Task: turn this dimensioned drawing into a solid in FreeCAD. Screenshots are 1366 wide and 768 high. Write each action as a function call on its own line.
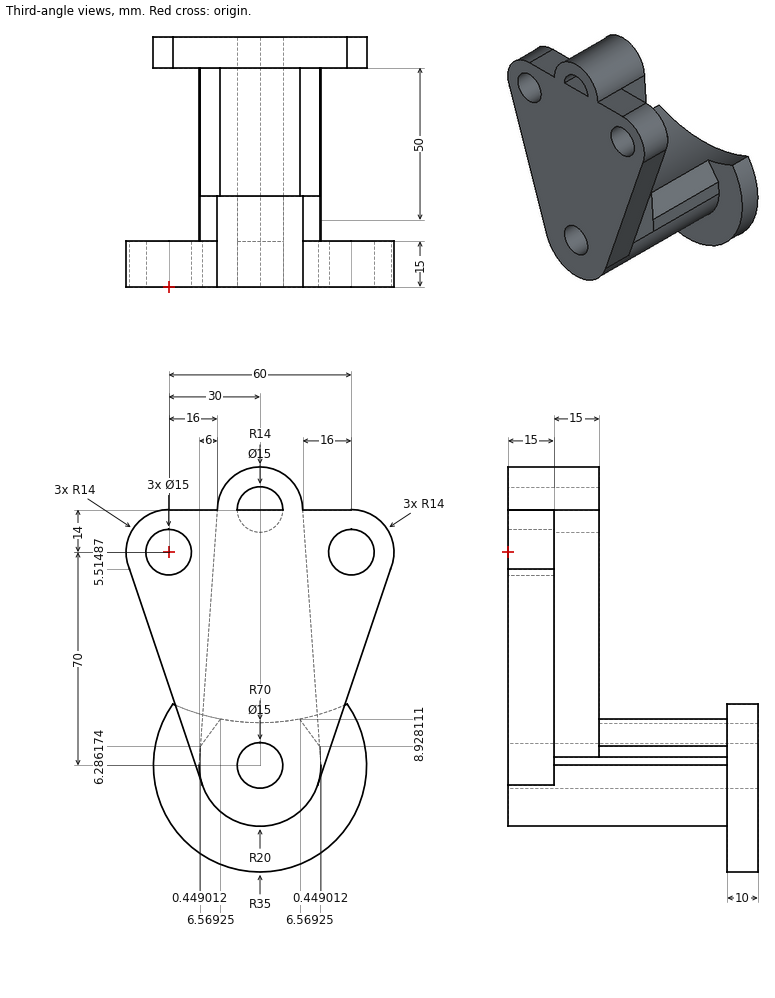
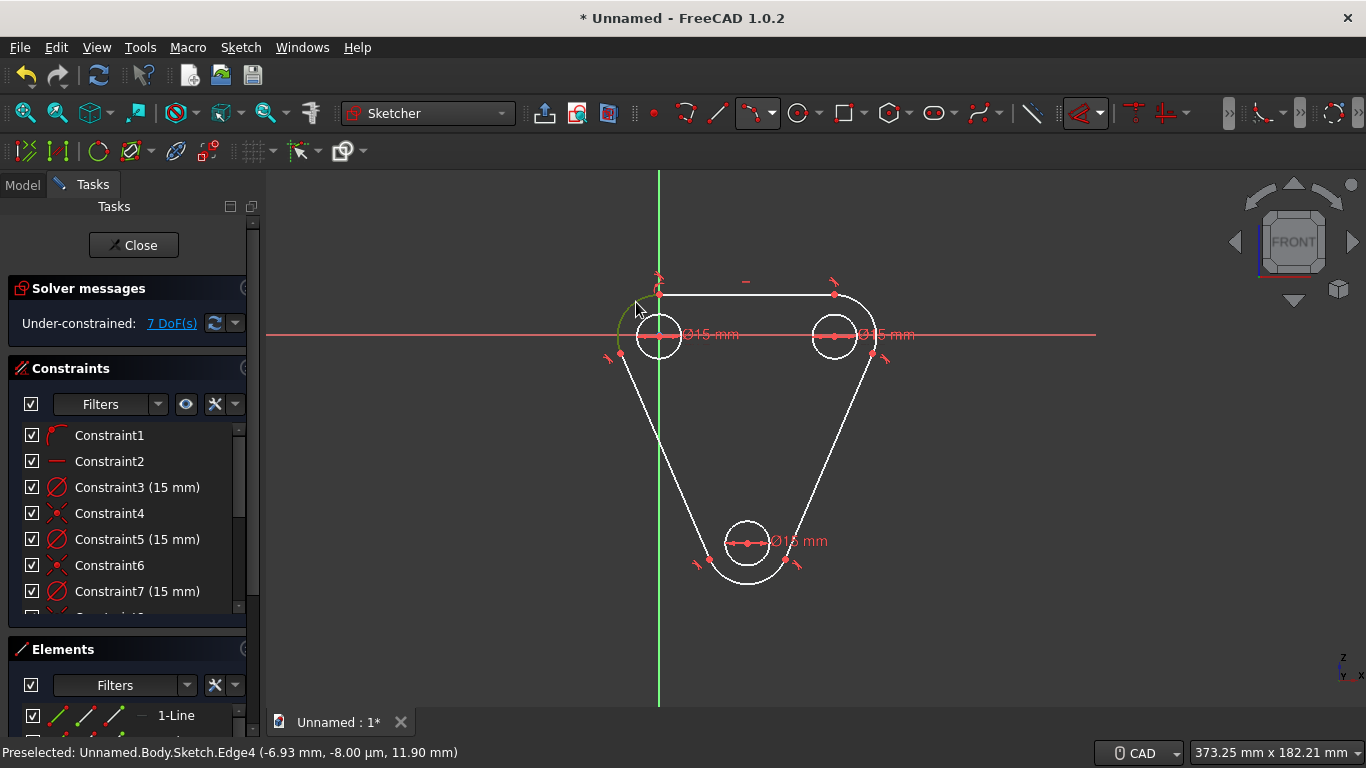
click(858, 302)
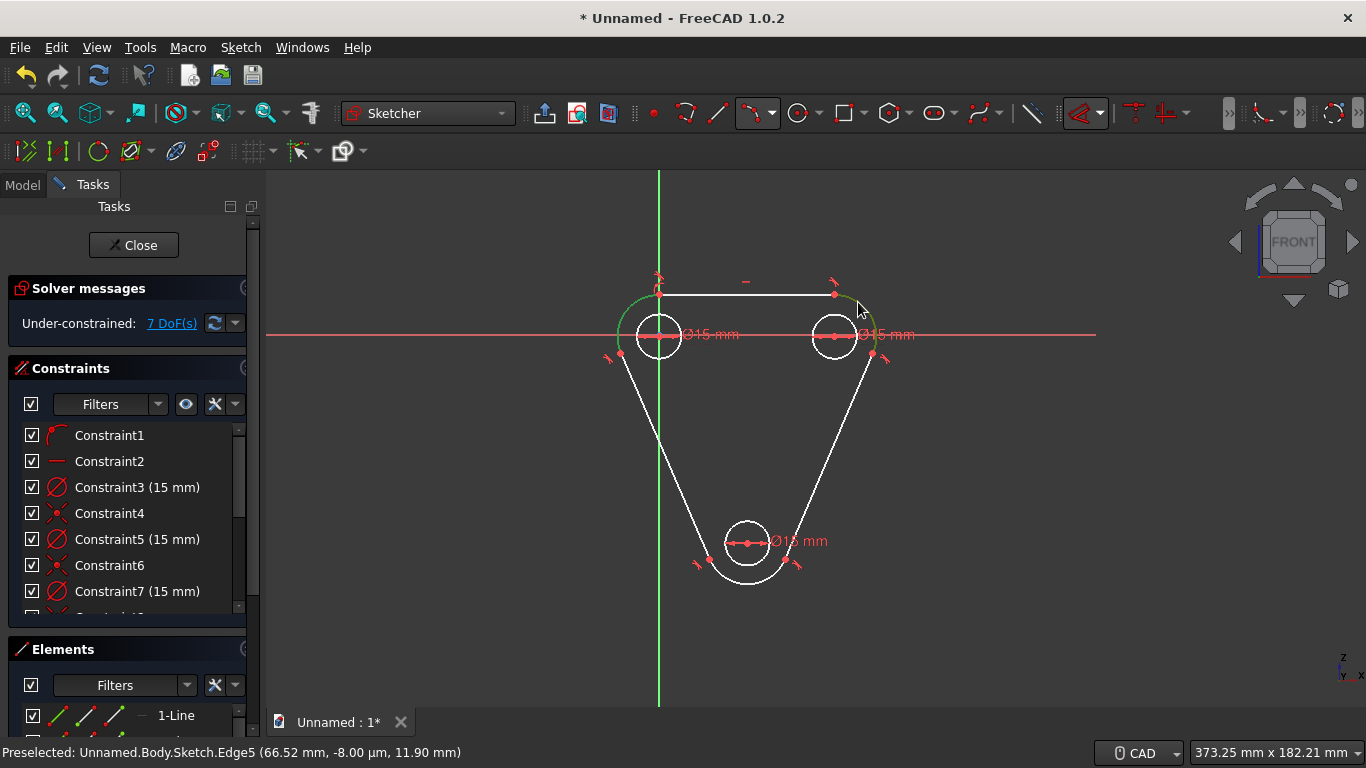
click(729, 580)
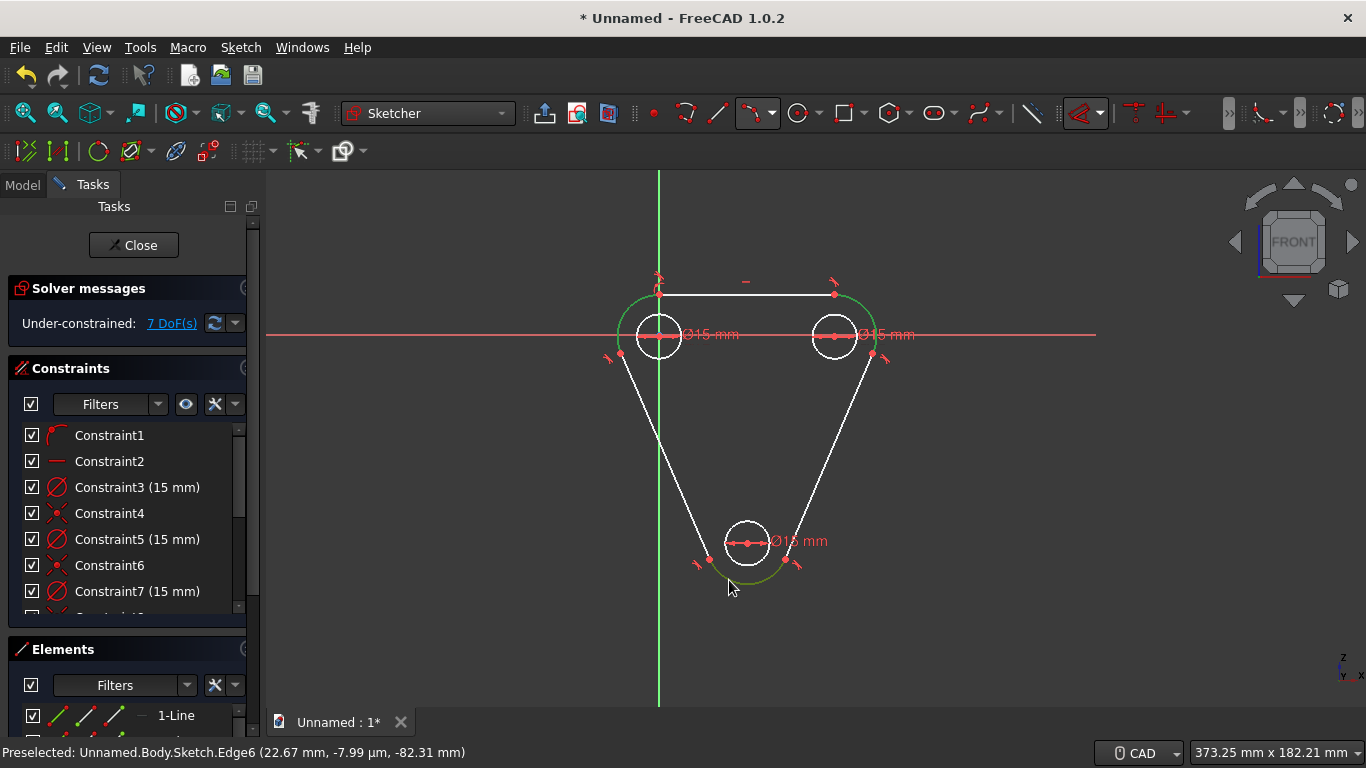
key(e)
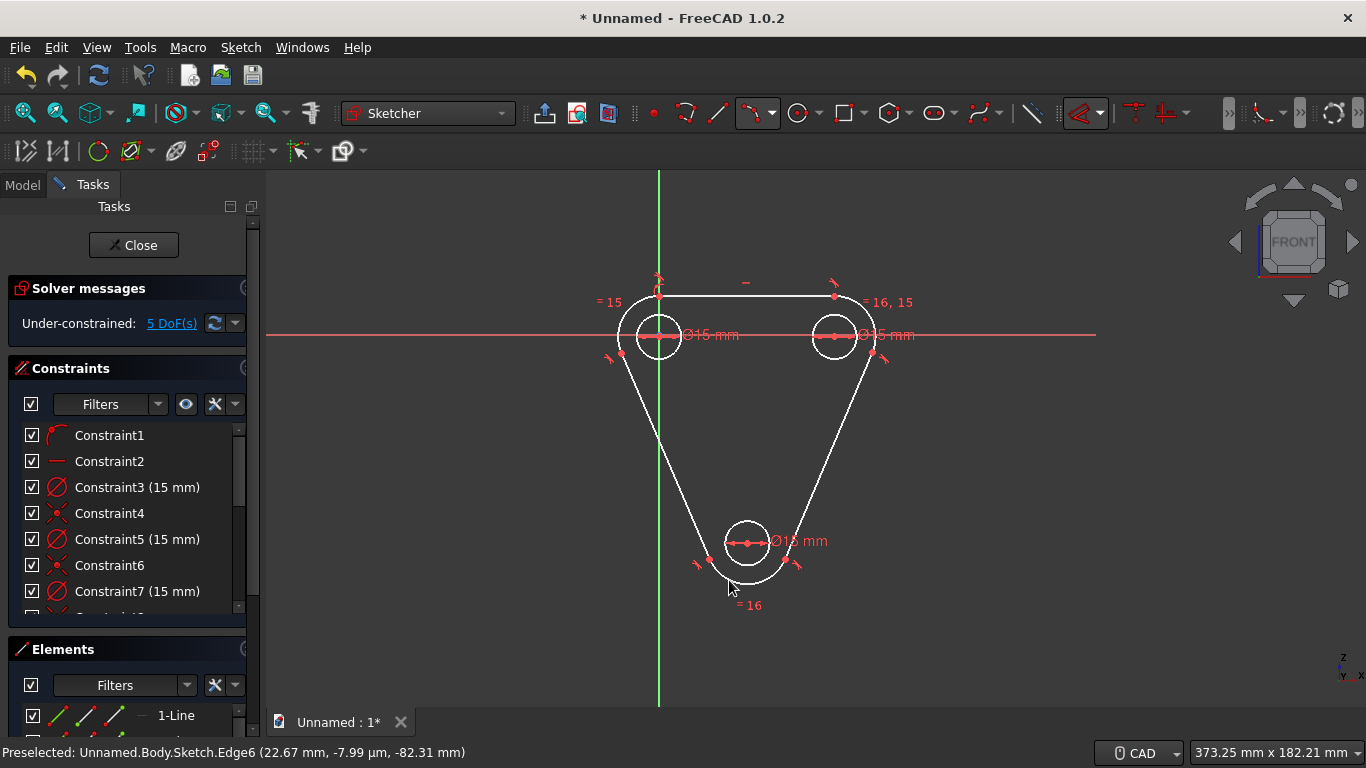
click(659, 337)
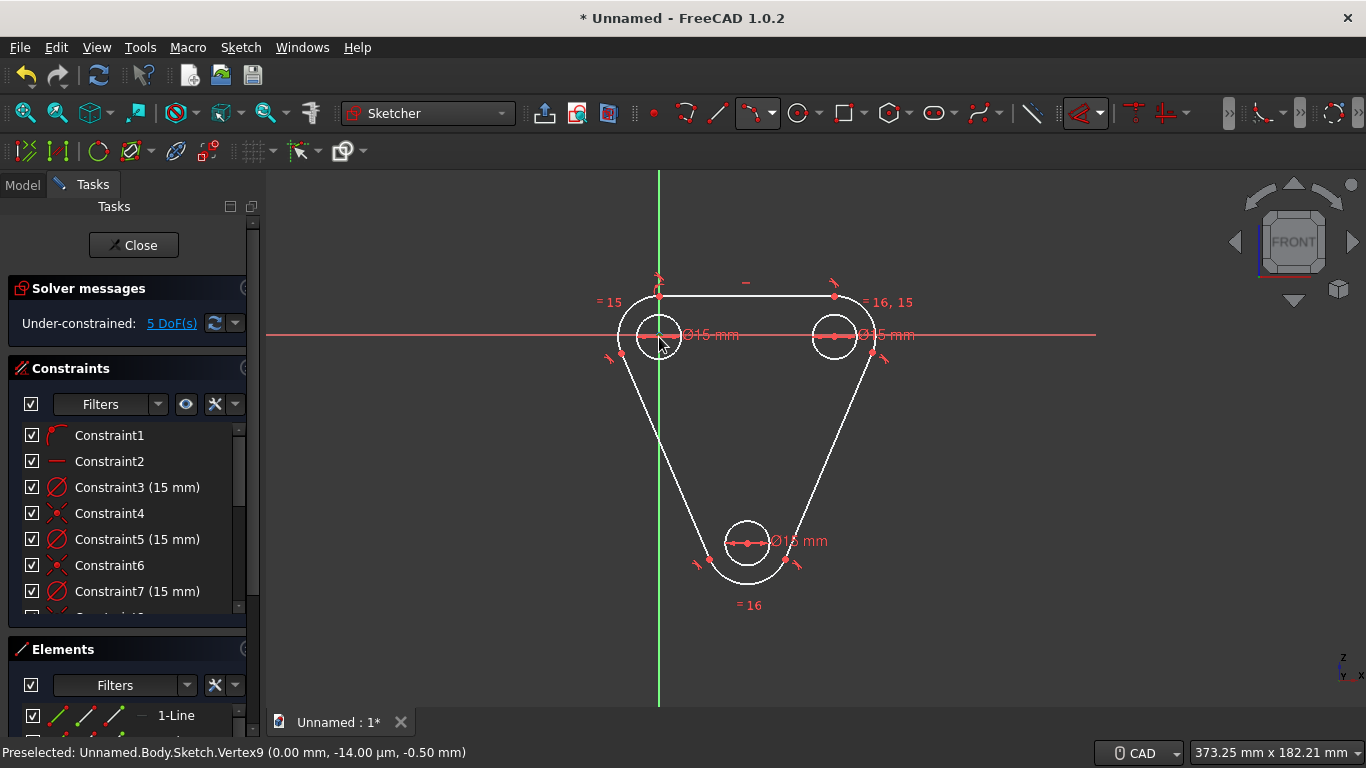
click(359, 335)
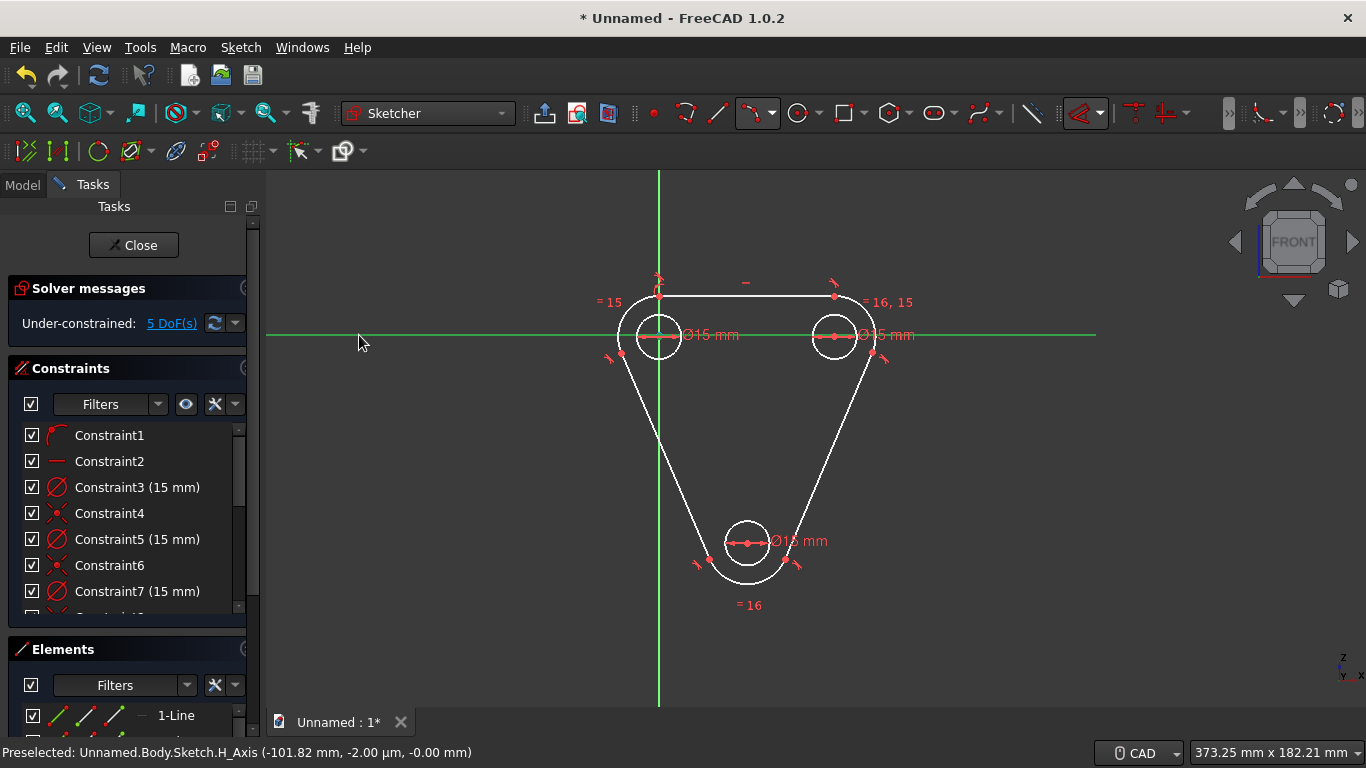
click(1134, 114)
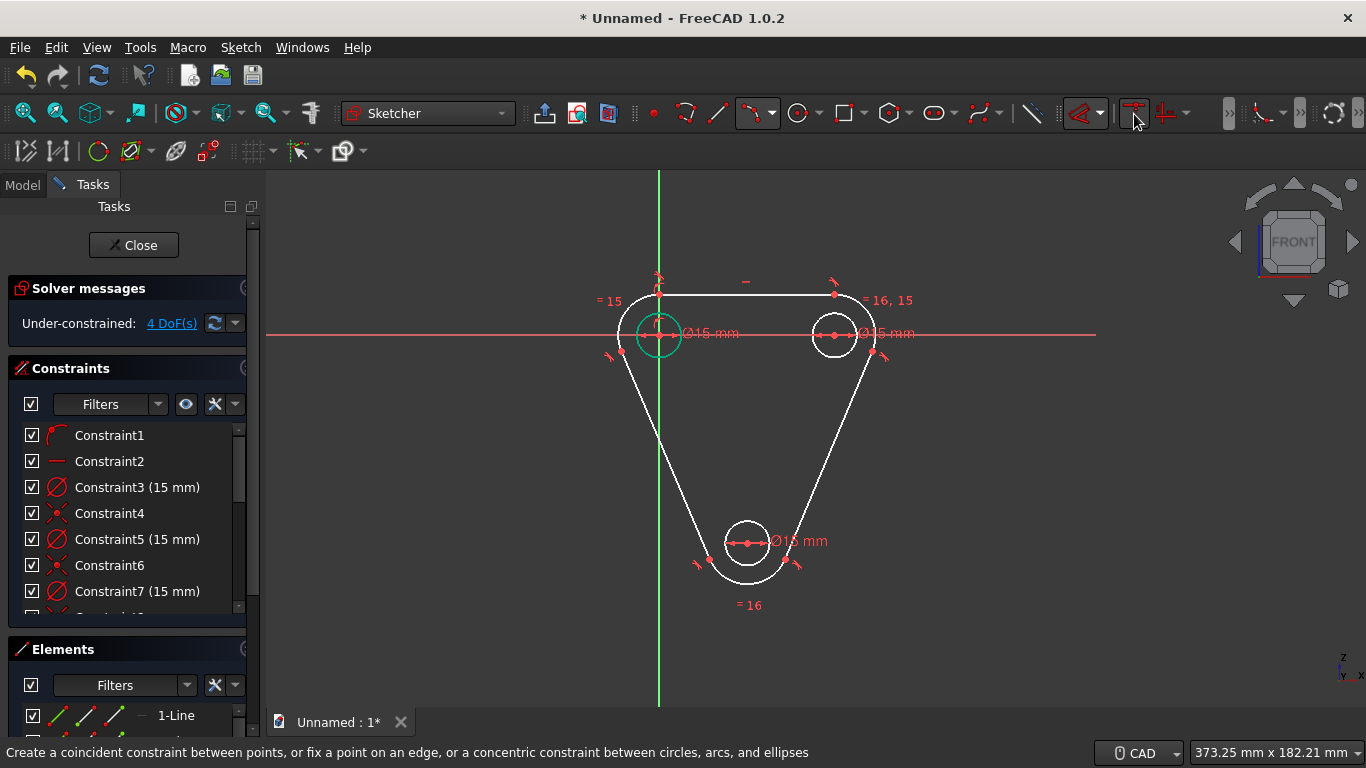
click(1080, 114)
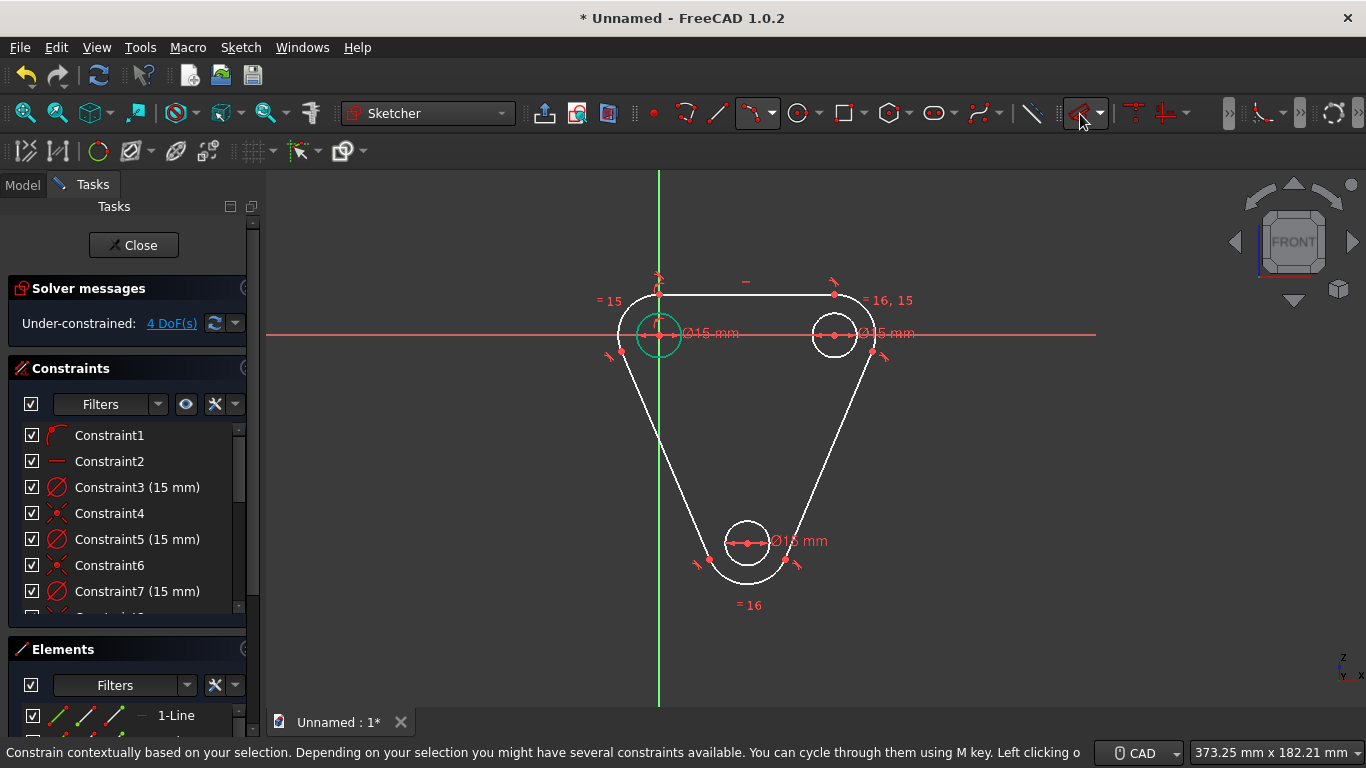
click(636, 302)
click(618, 276)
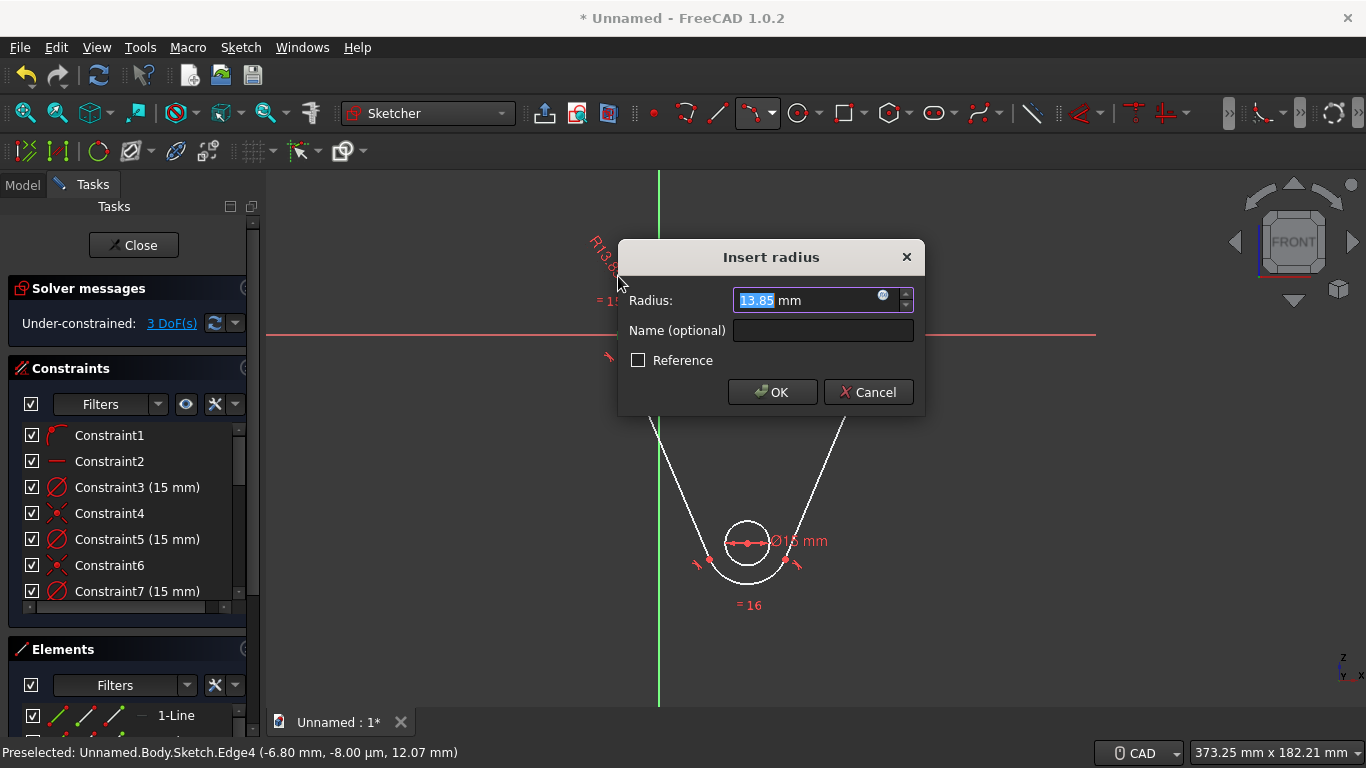
text(14)
key(Return)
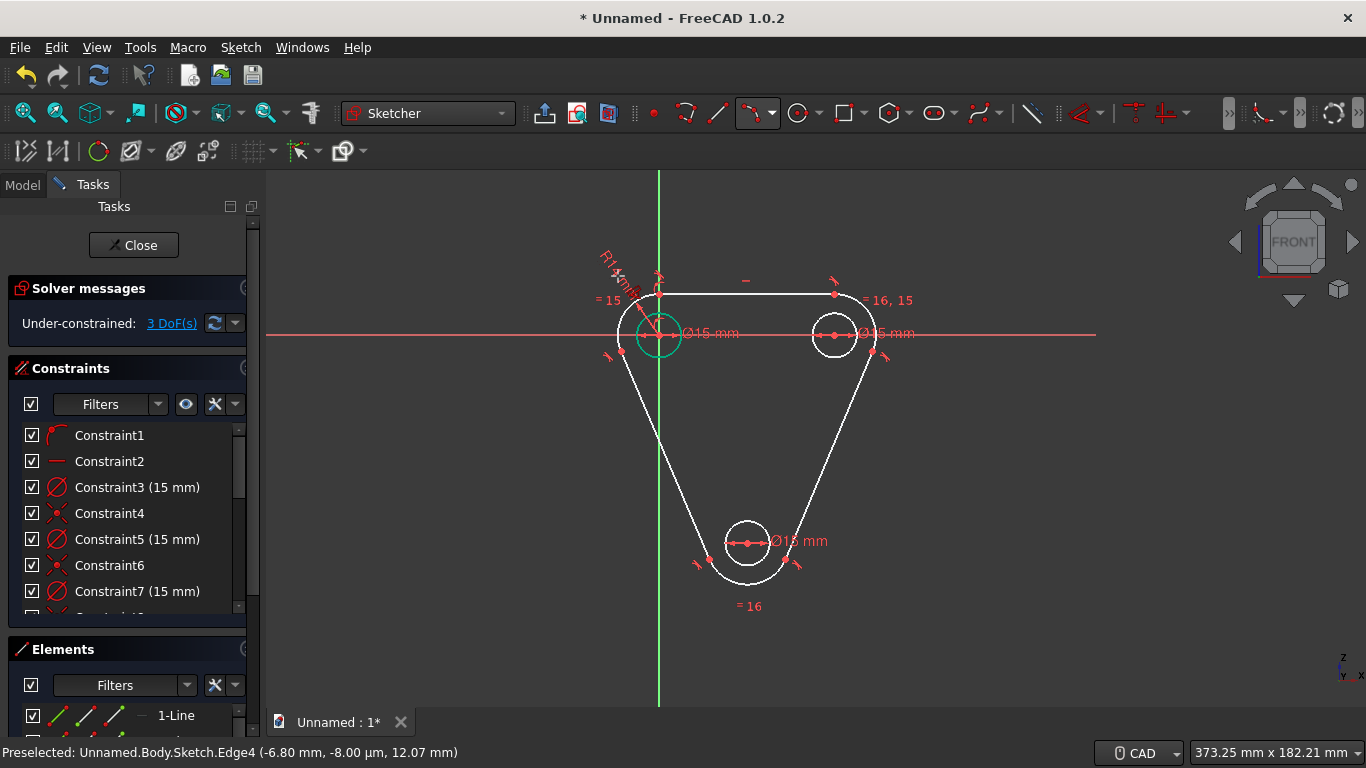
click(712, 294)
click(747, 260)